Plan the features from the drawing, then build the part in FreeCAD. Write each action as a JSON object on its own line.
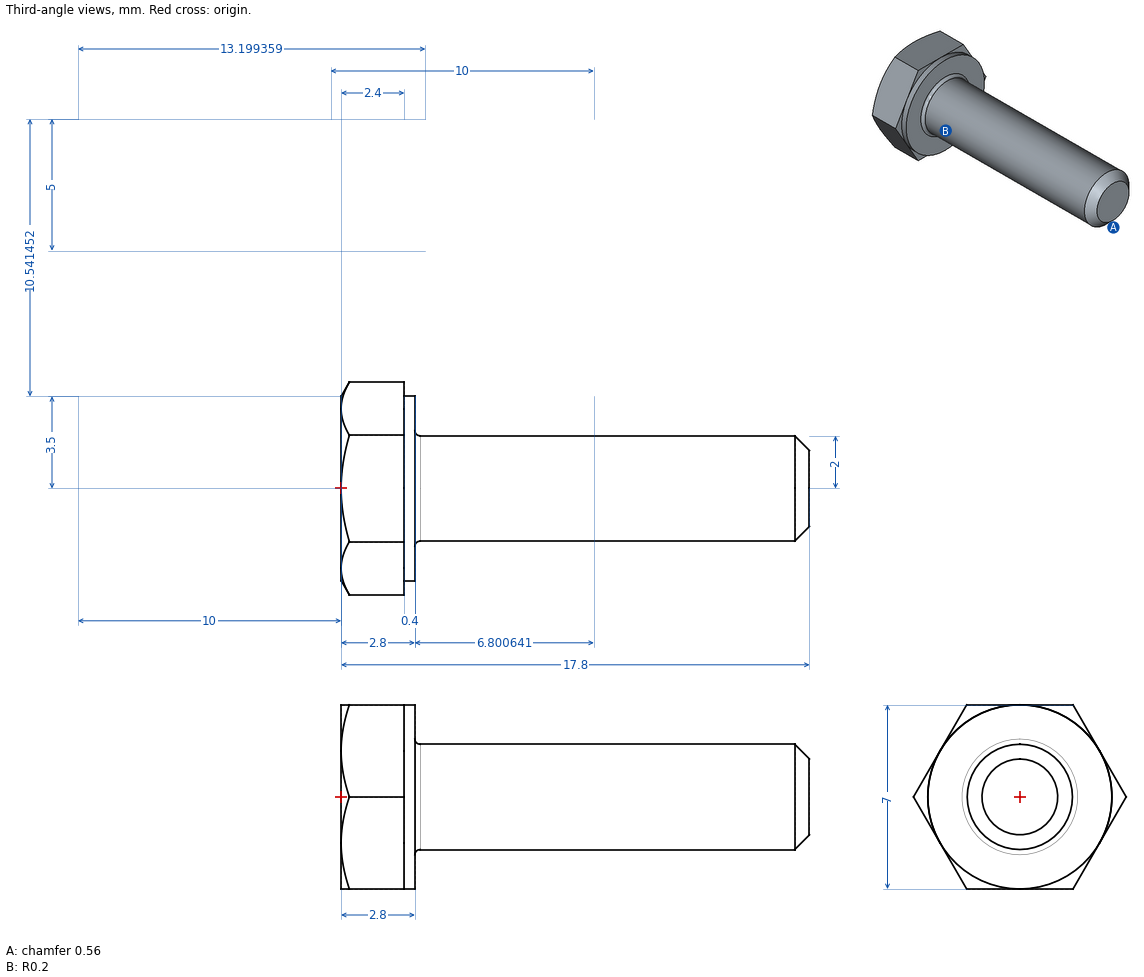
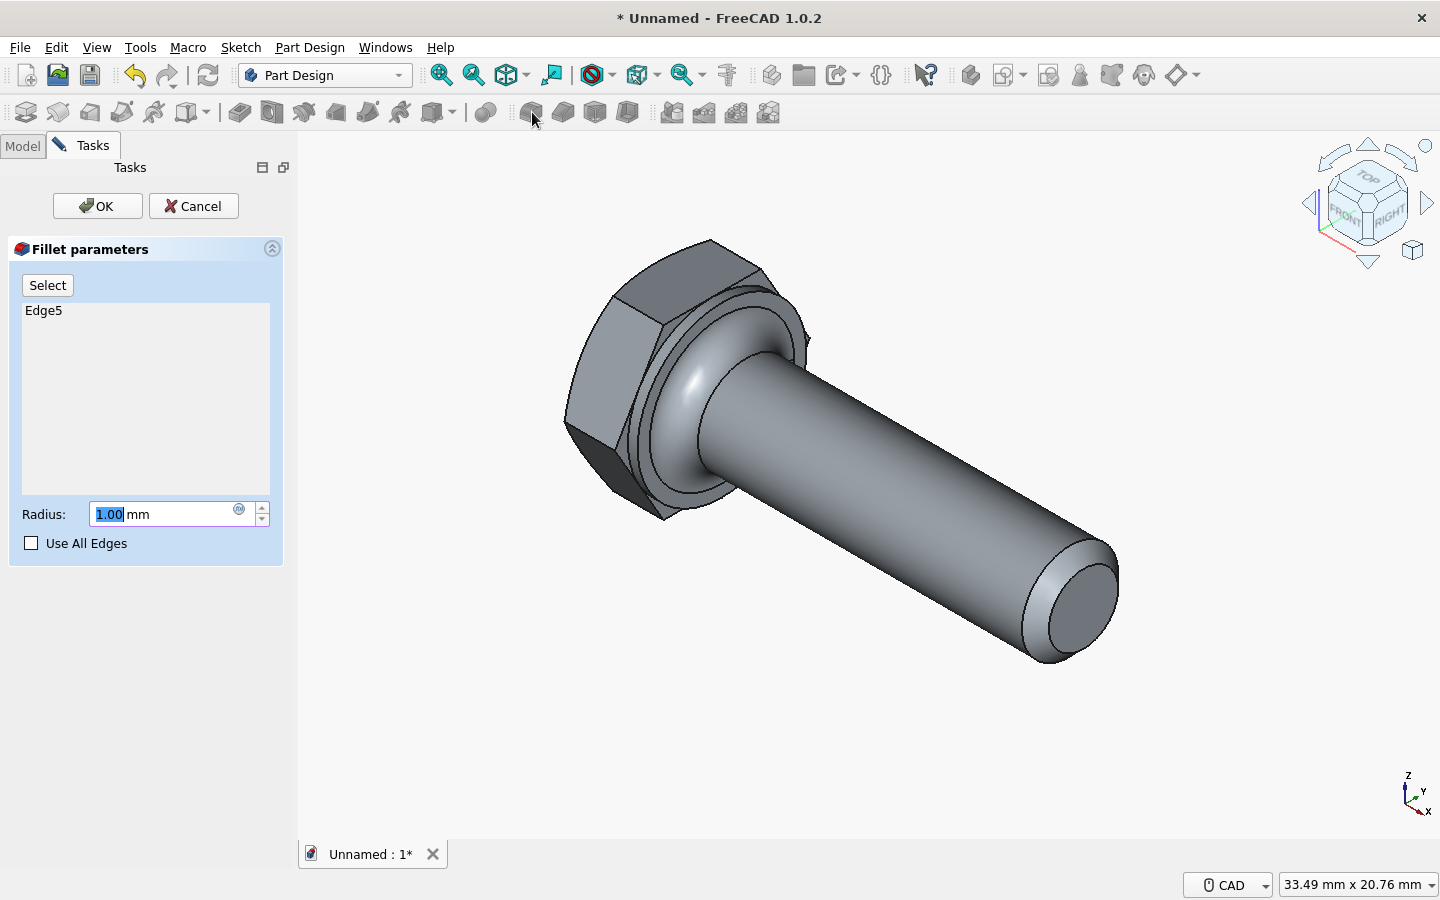
{"action": "type", "text": "0.2"}
{"action": "key", "text": "Tab"}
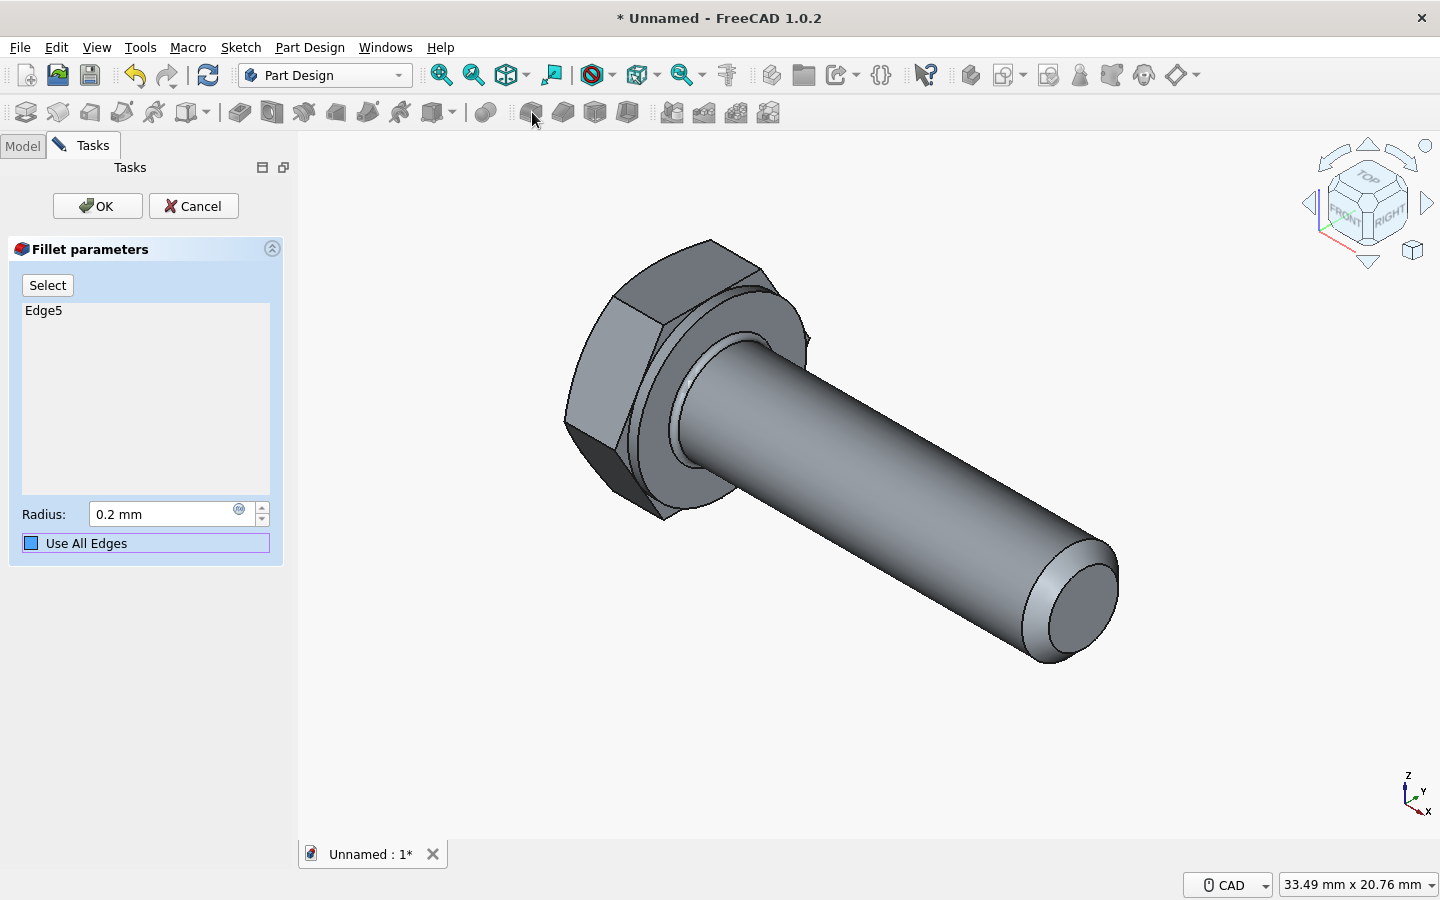
{"action": "left_click", "coordinate": [98, 206]}